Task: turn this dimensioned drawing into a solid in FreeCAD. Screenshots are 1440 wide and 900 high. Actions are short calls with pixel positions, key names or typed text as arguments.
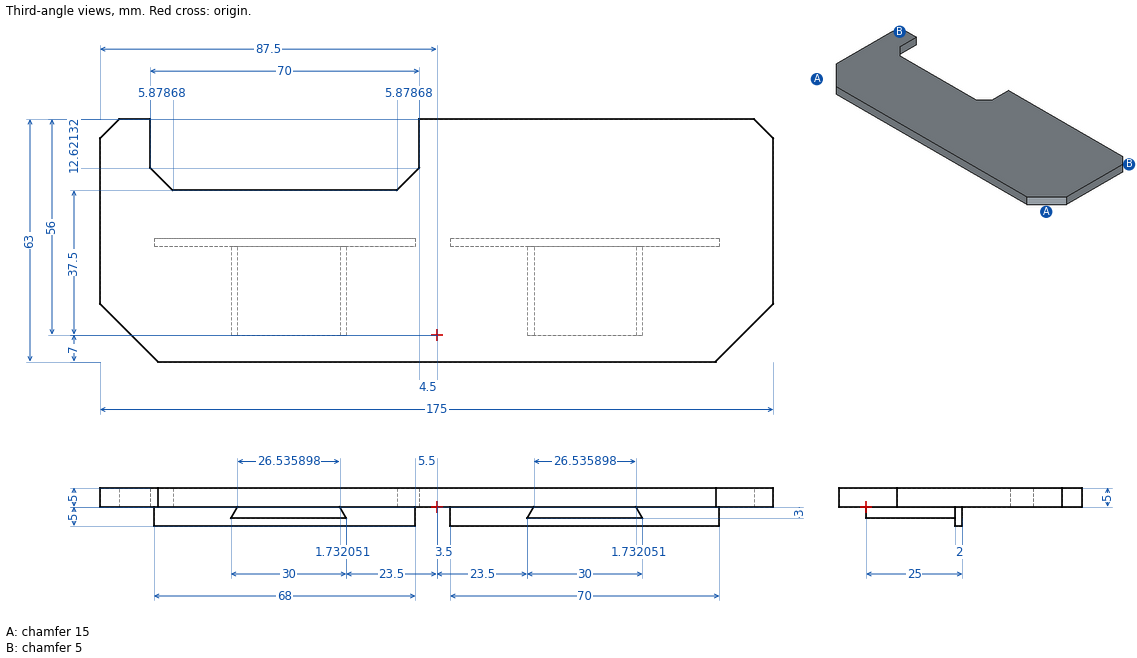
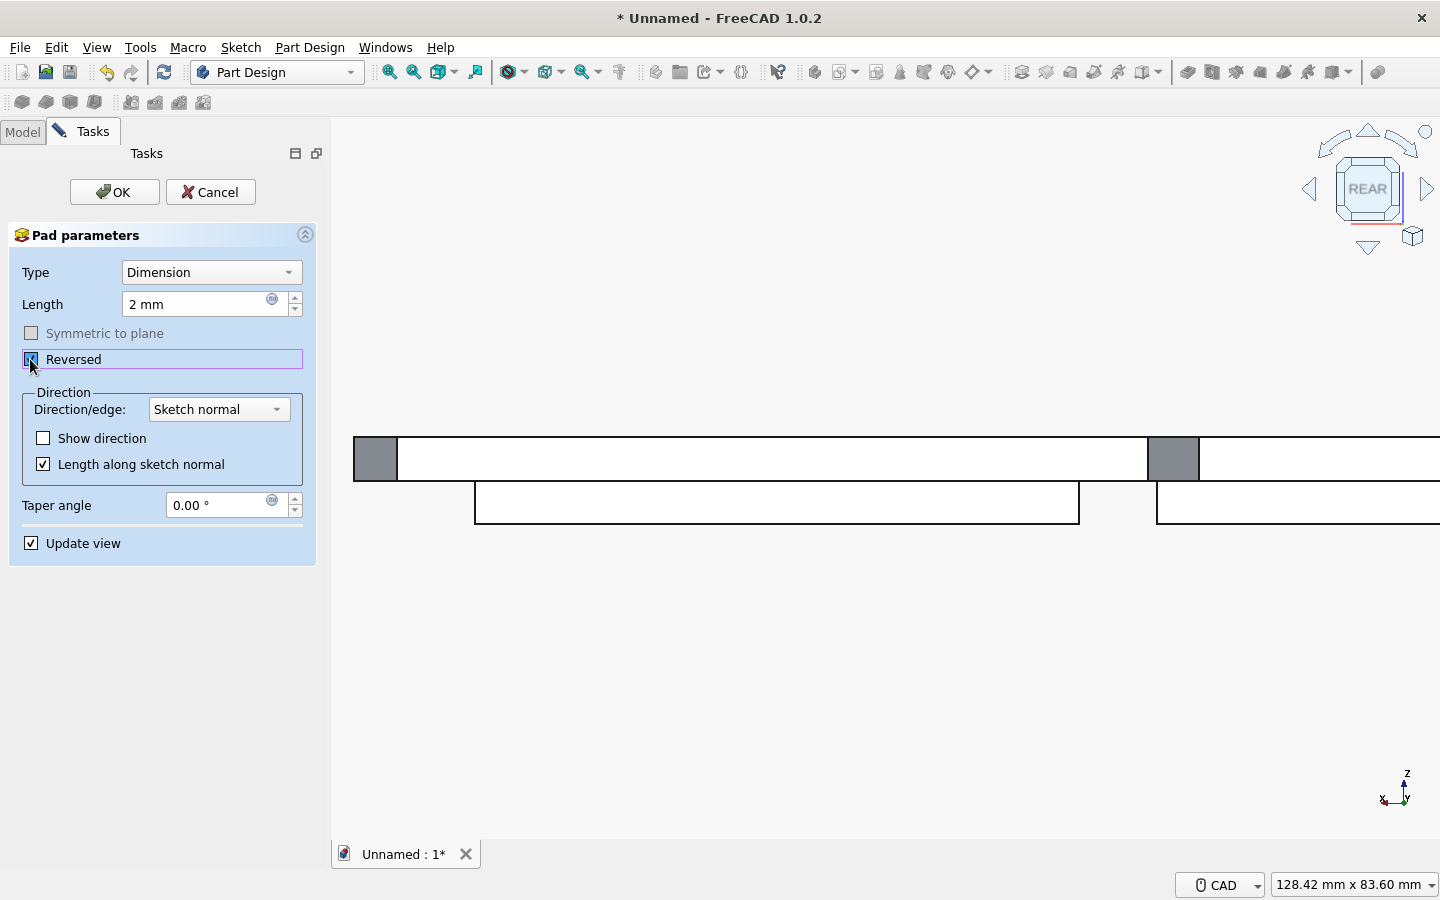
click(115, 192)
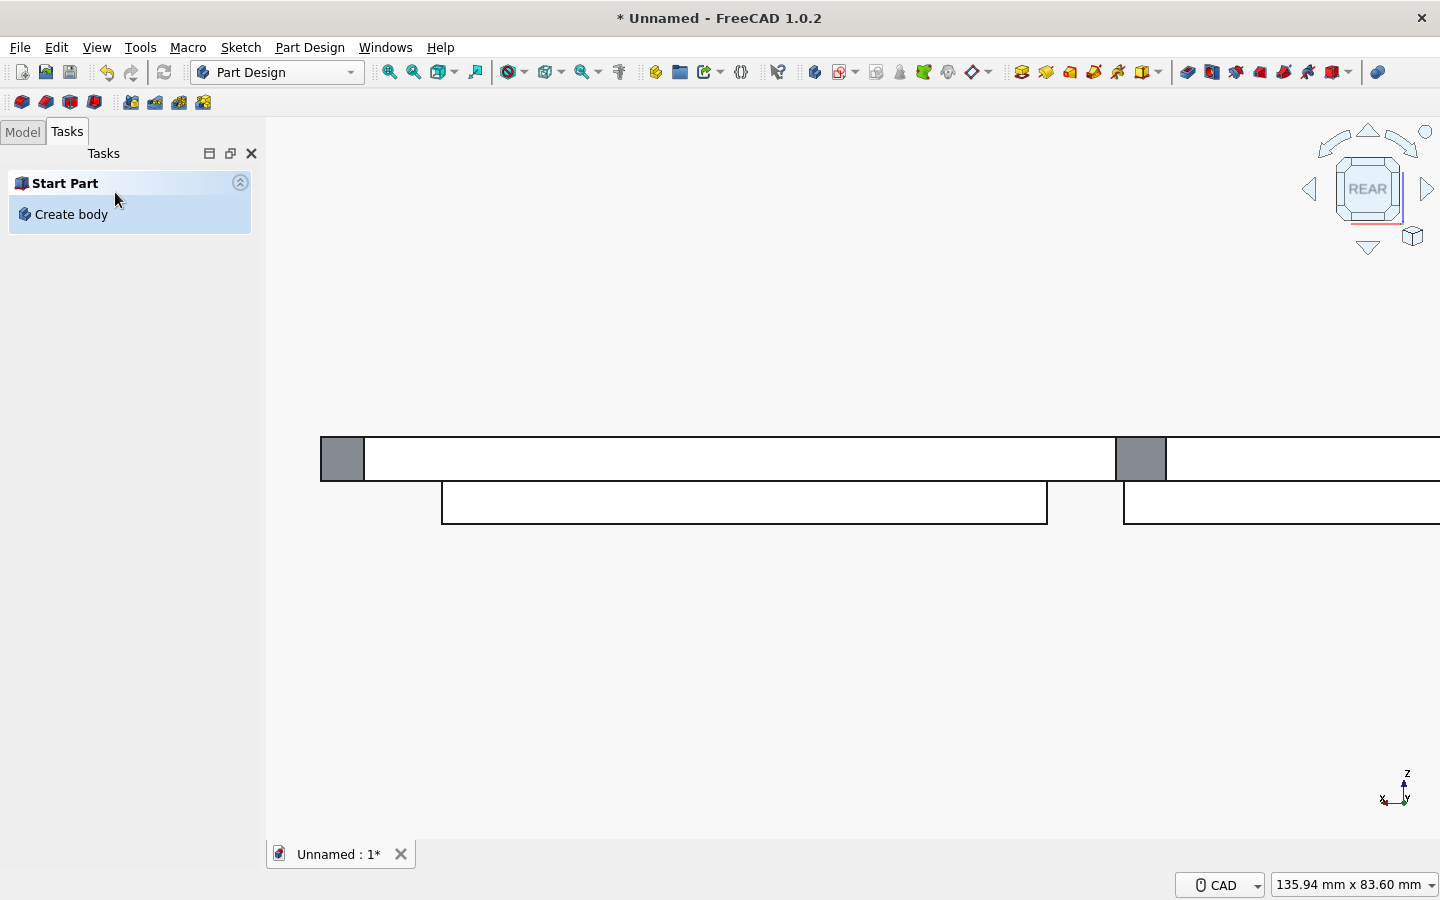
key(0)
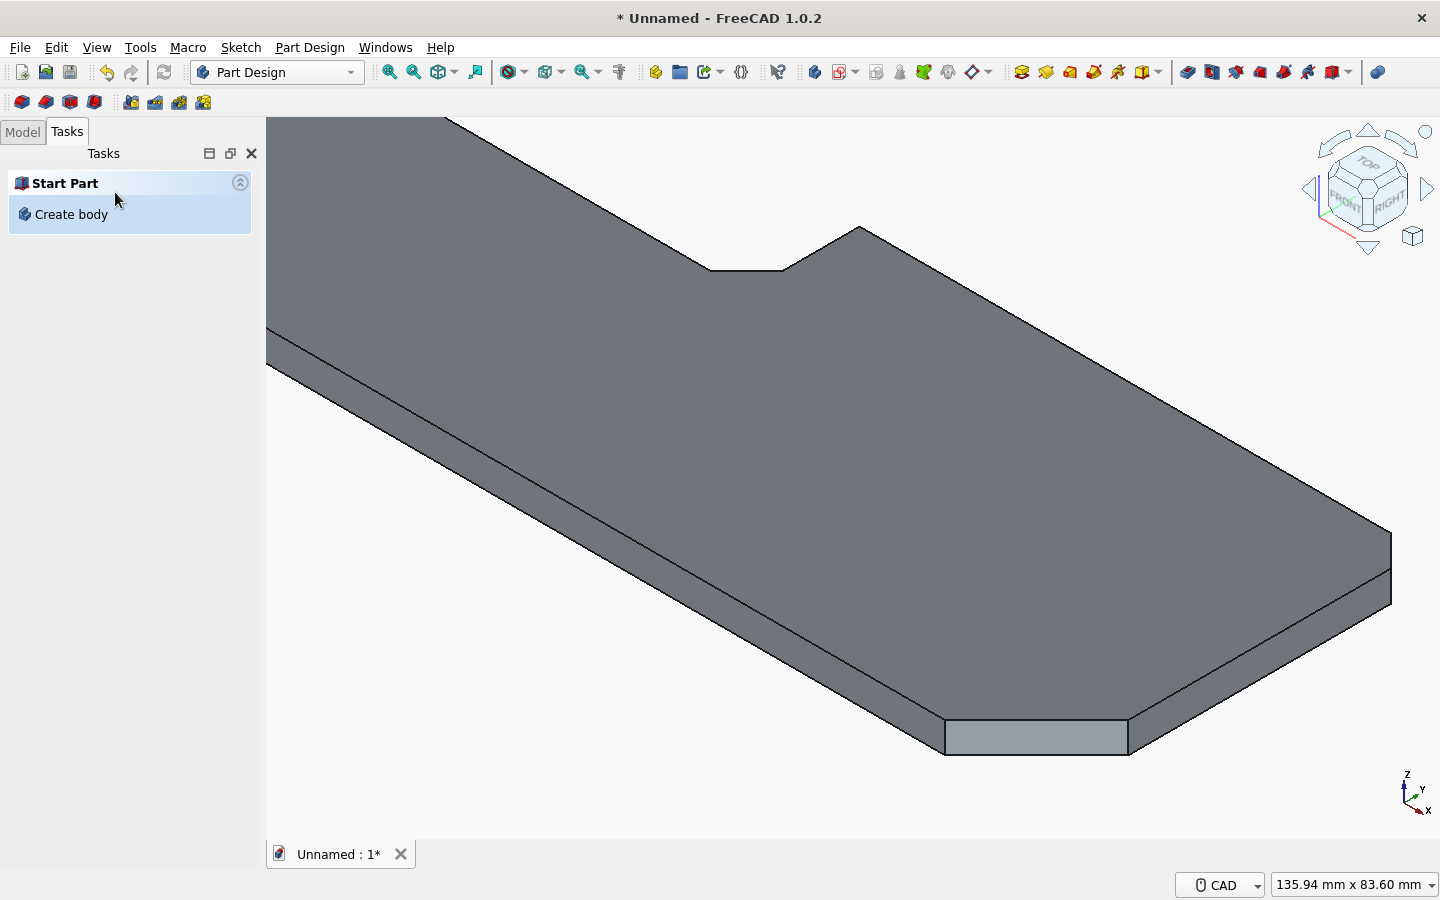
click(390, 72)